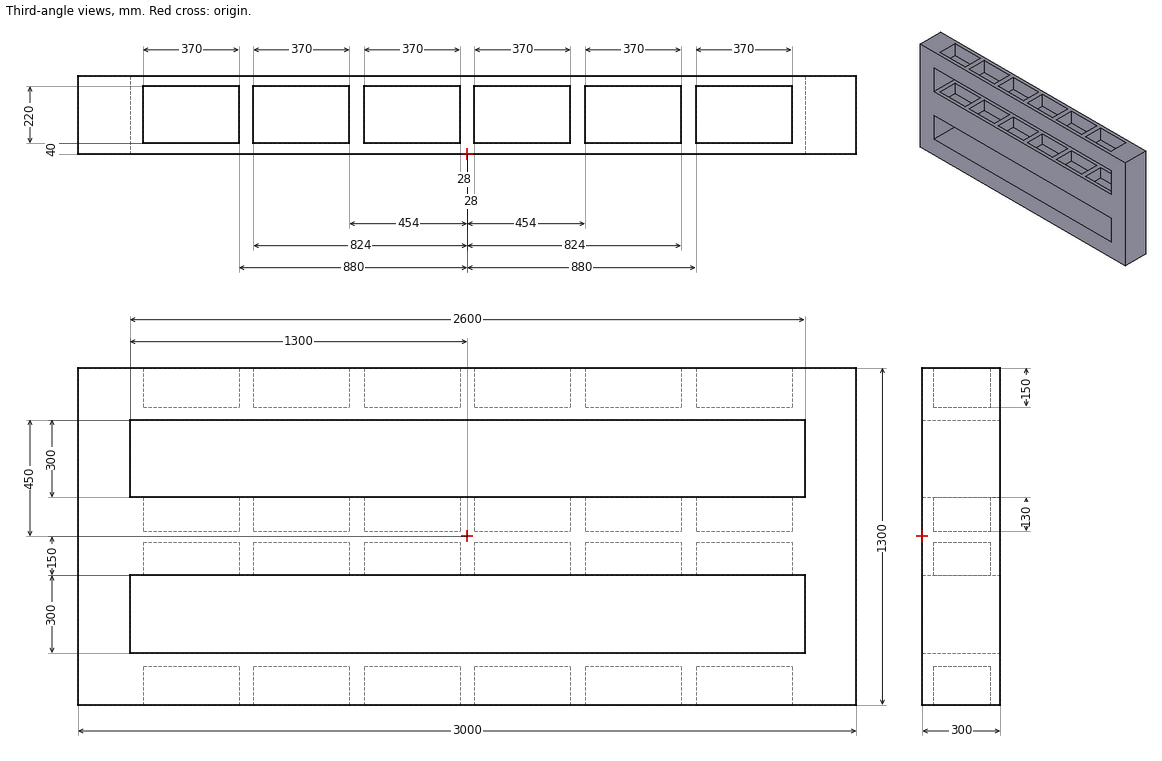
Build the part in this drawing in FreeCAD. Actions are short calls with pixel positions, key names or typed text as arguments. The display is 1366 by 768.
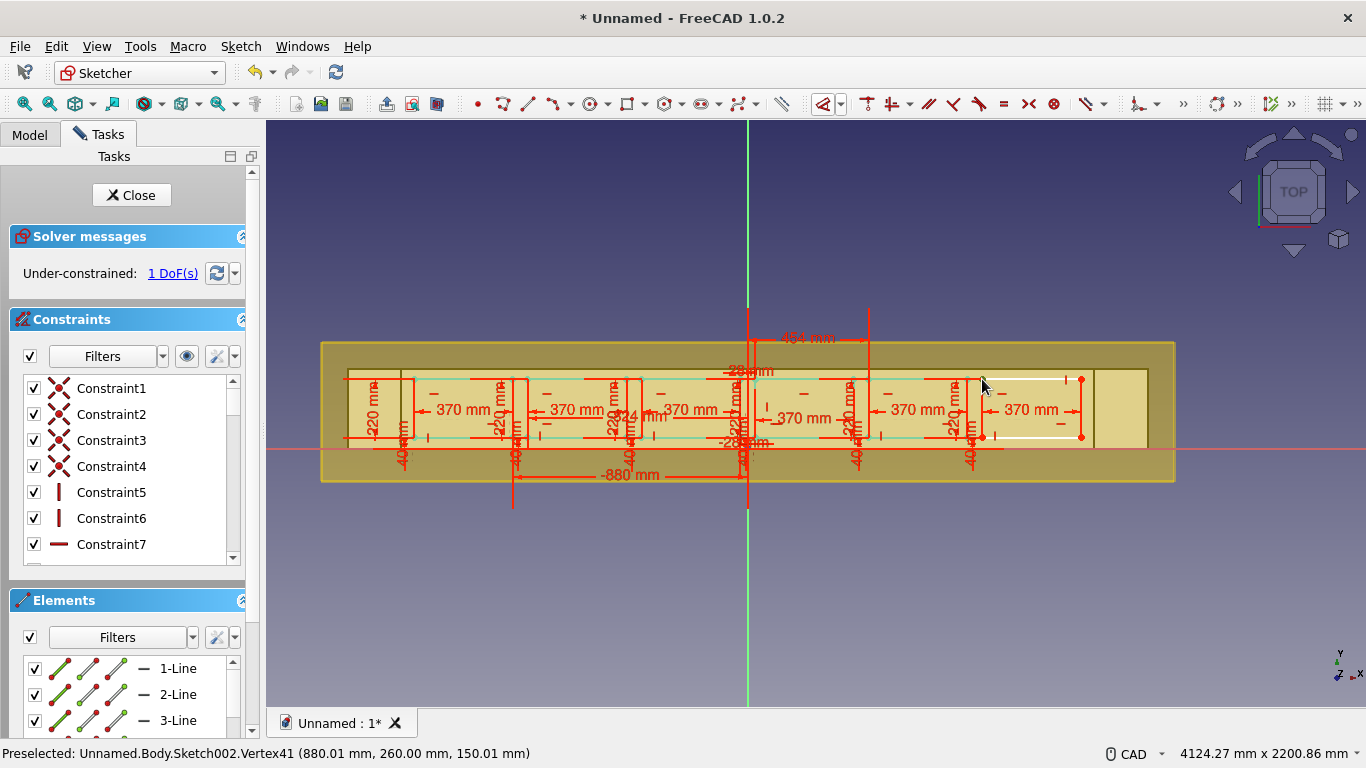
key(l)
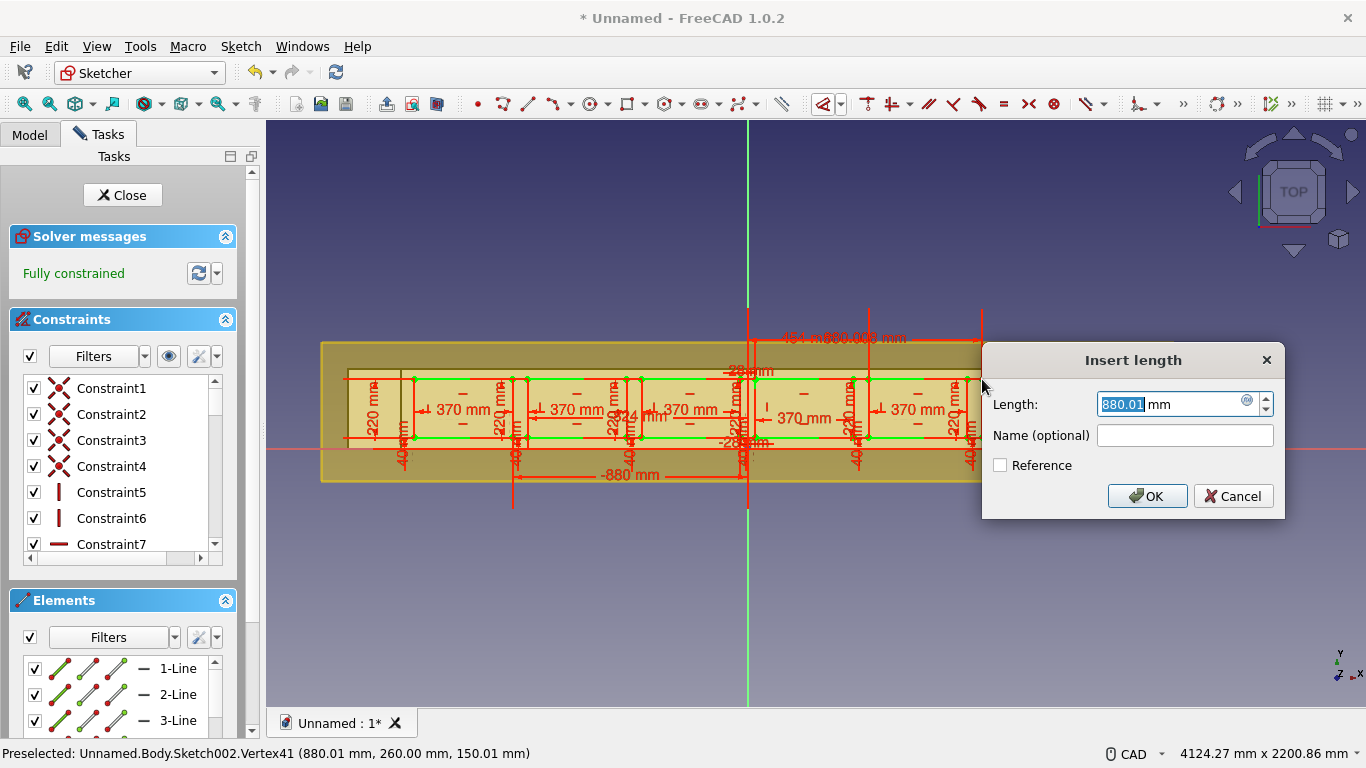
text(880)
key(Return)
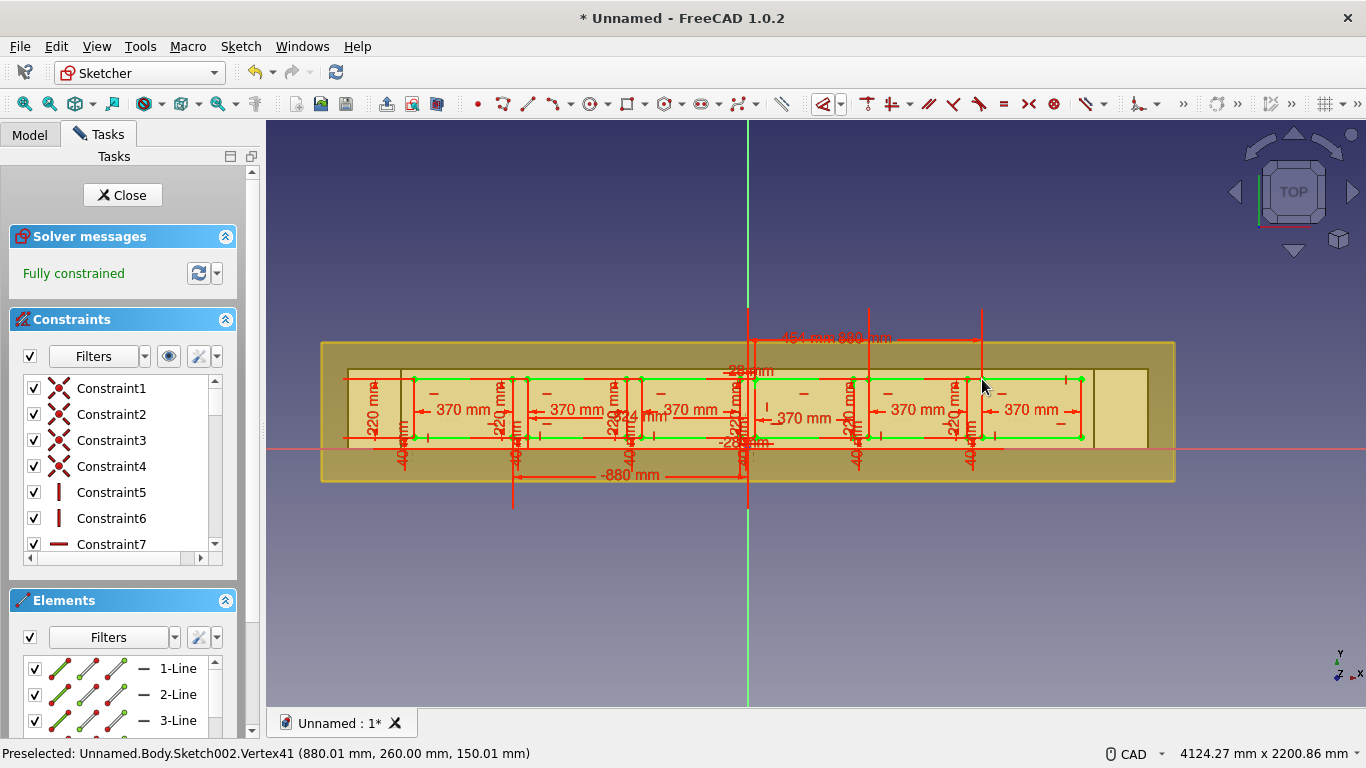
click(123, 195)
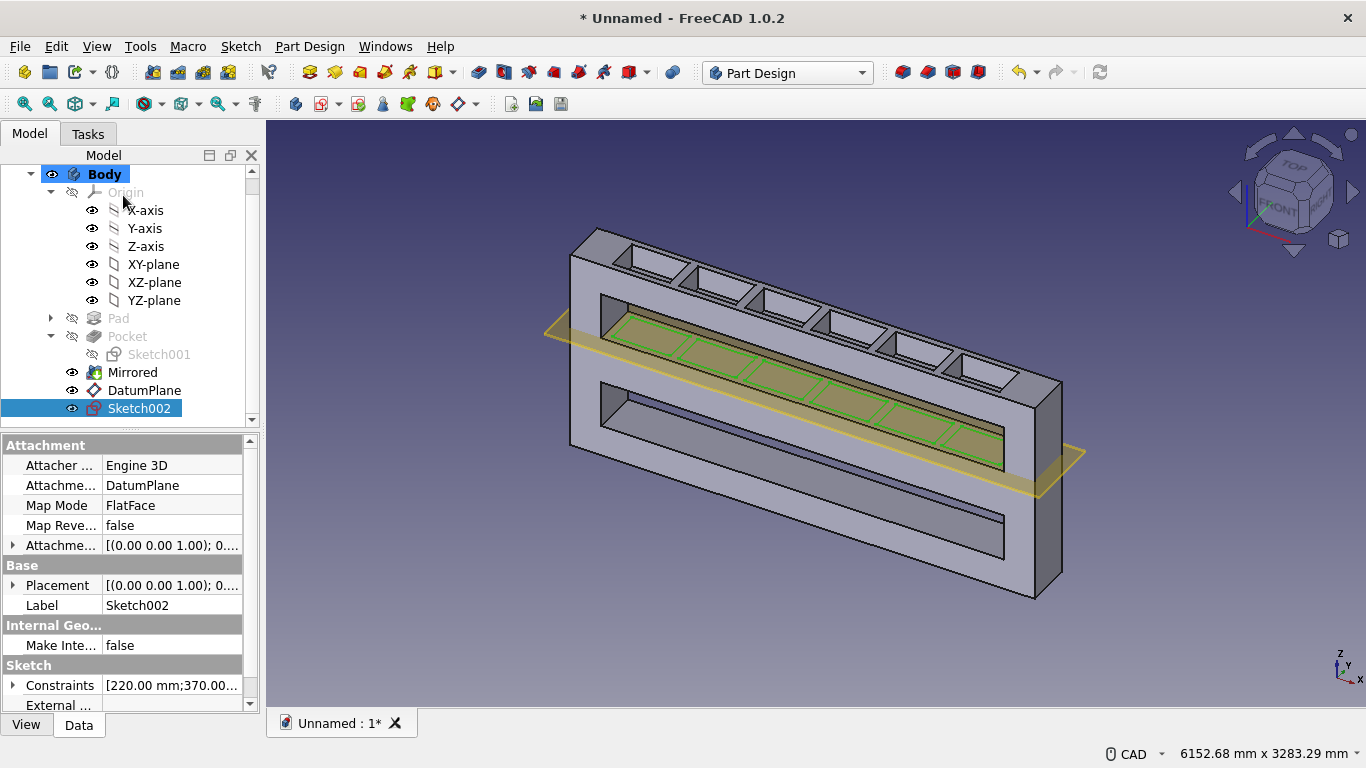
click(479, 72)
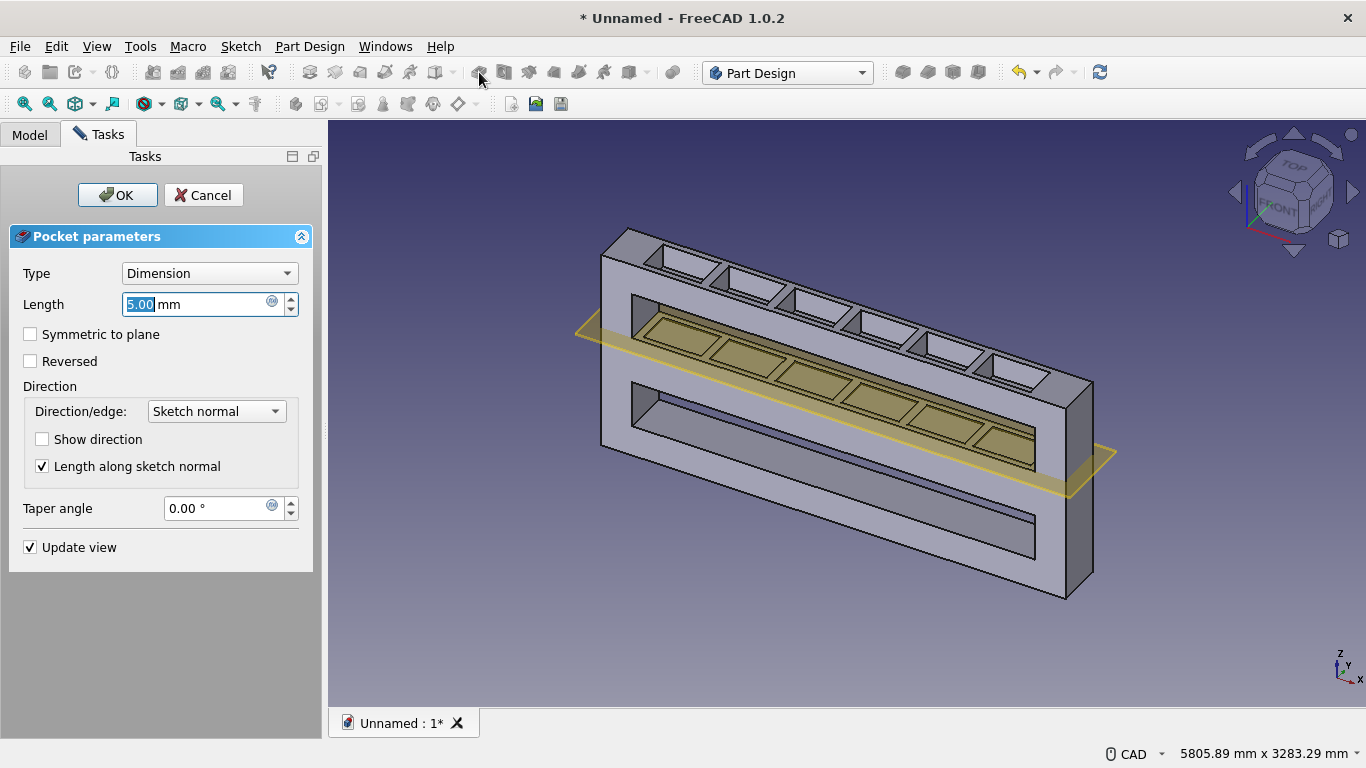
text(130)
key(Tab)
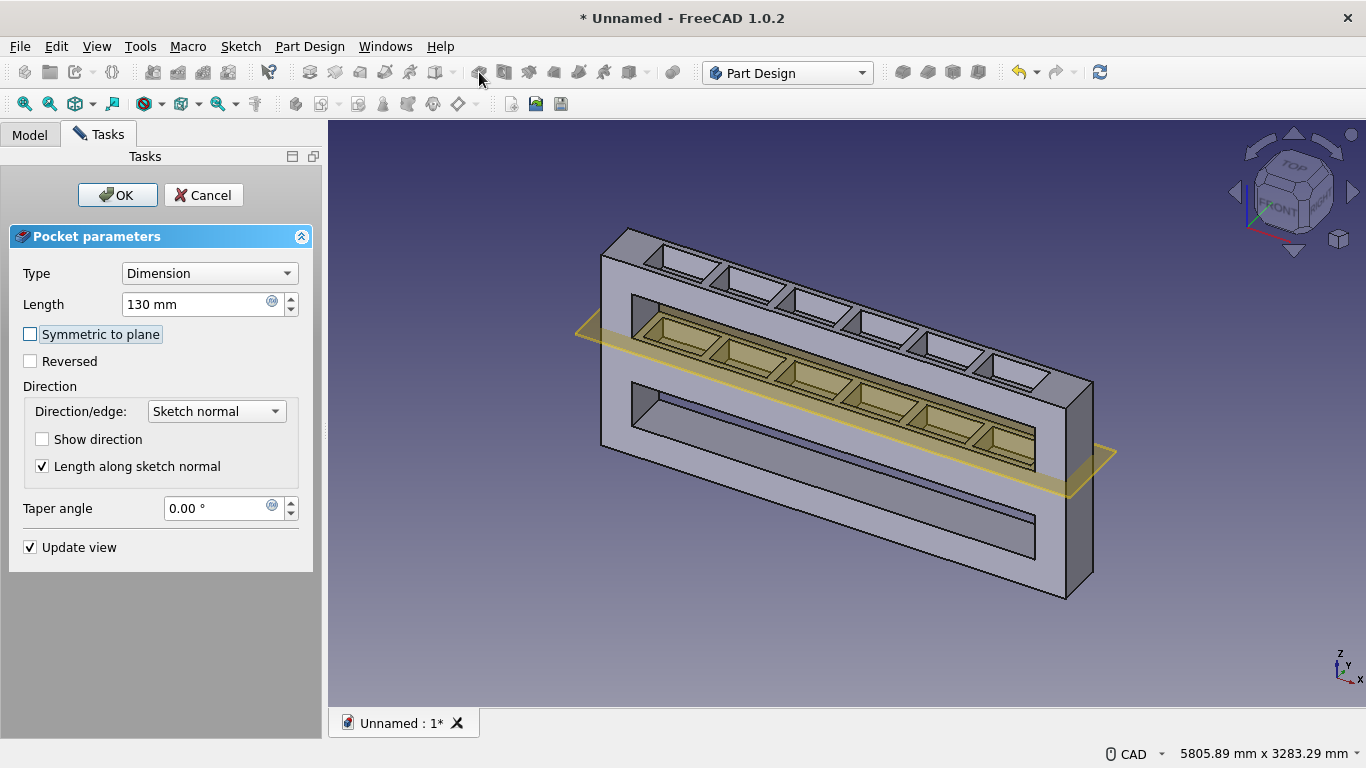
click(118, 195)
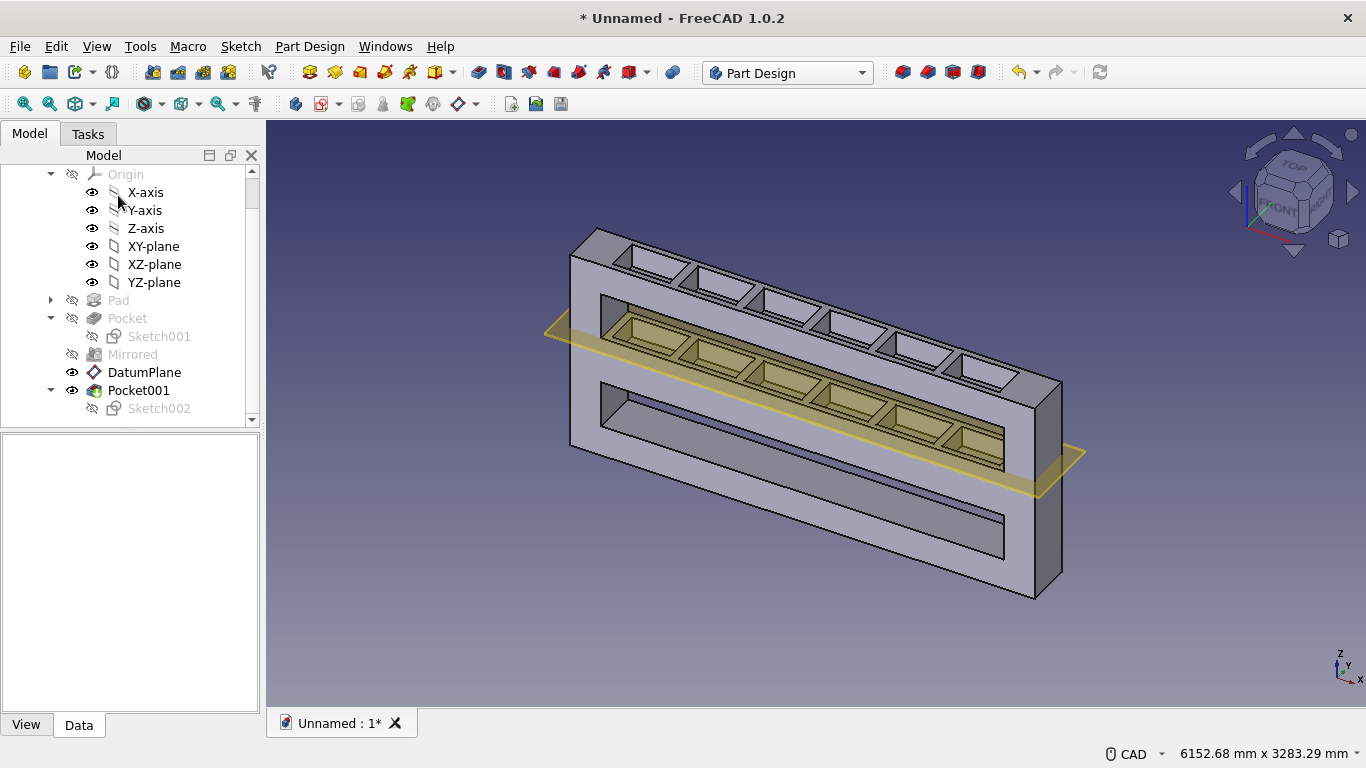
click(117, 372)
key(space)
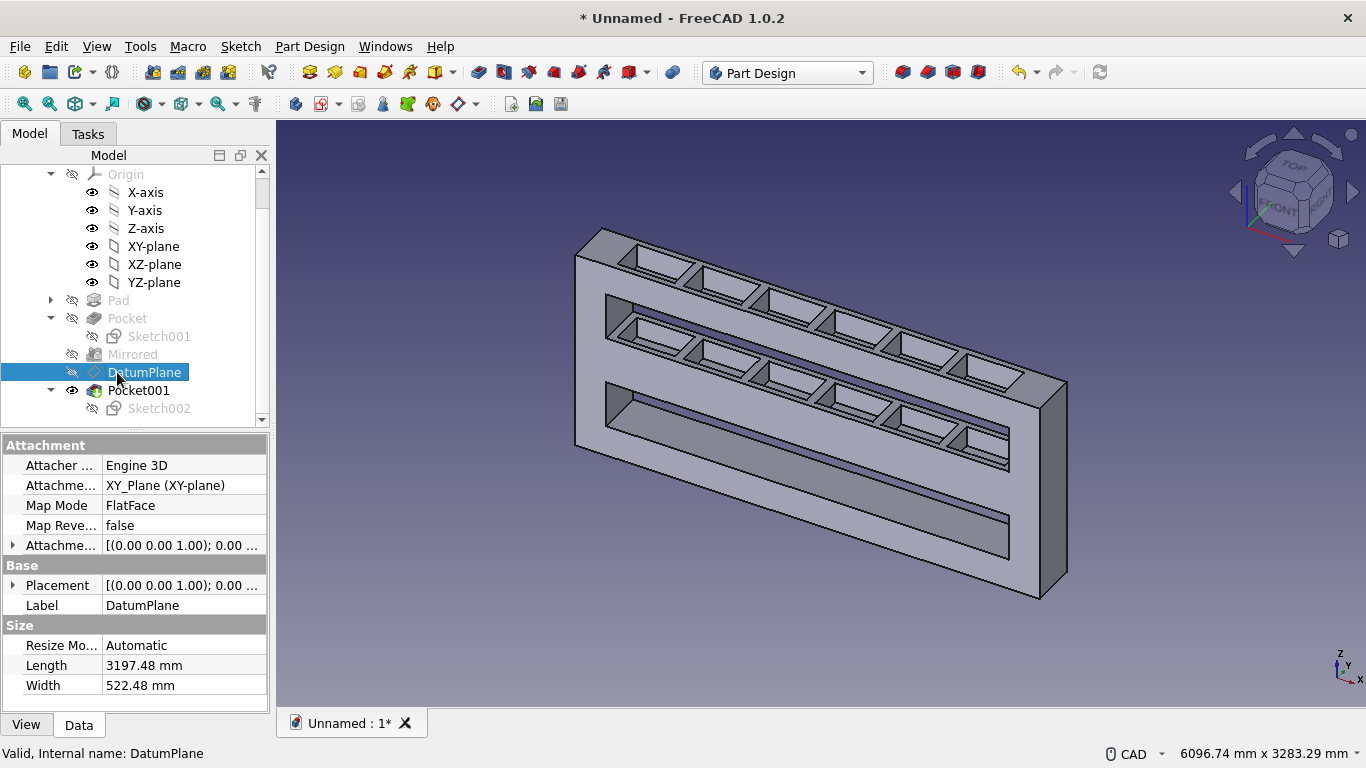
click(117, 390)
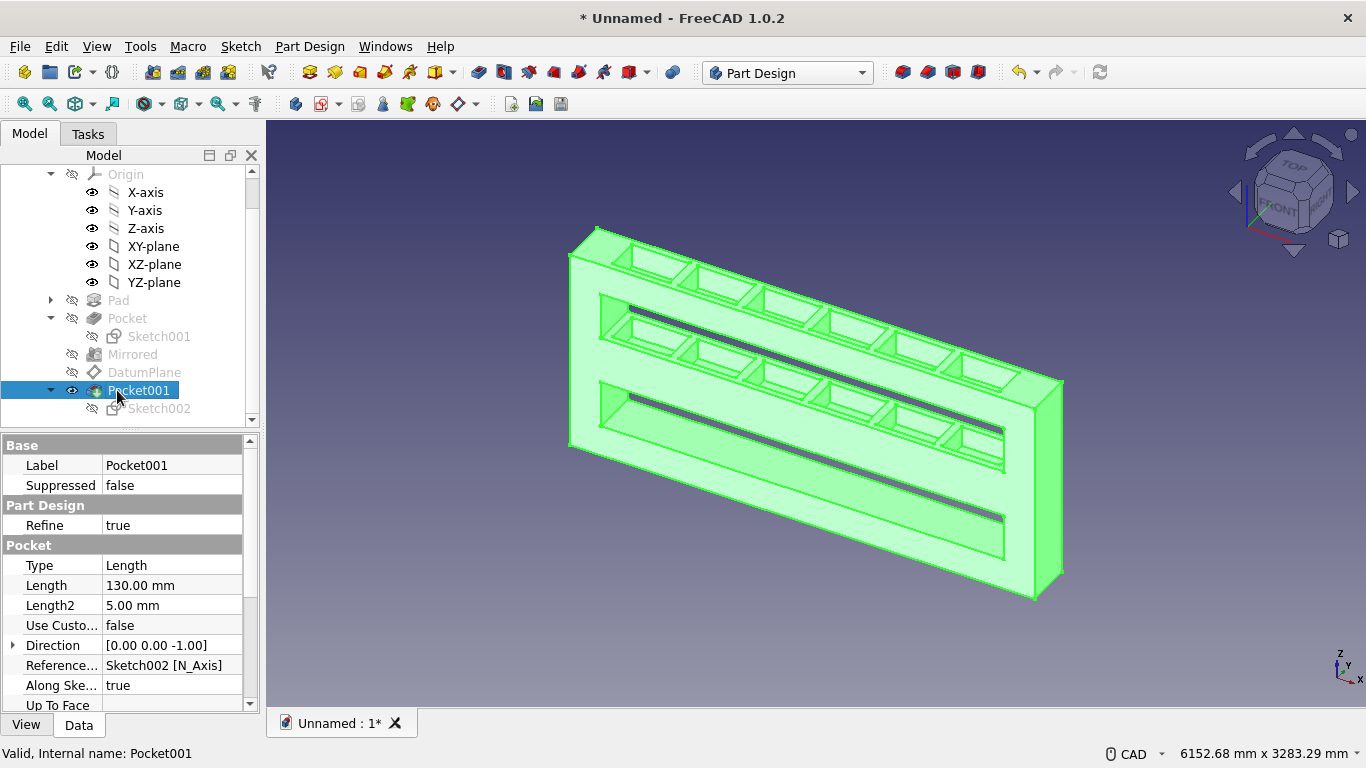
click(153, 72)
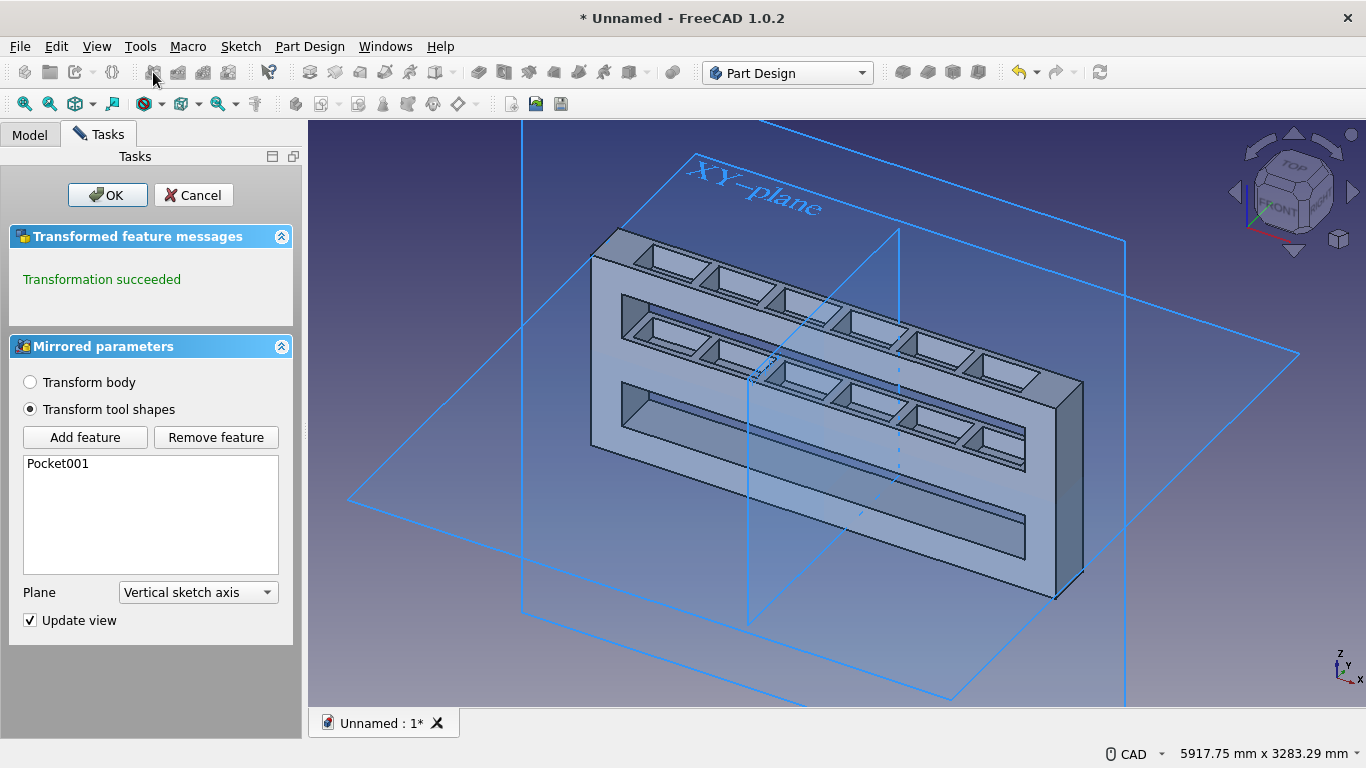
click(199, 592)